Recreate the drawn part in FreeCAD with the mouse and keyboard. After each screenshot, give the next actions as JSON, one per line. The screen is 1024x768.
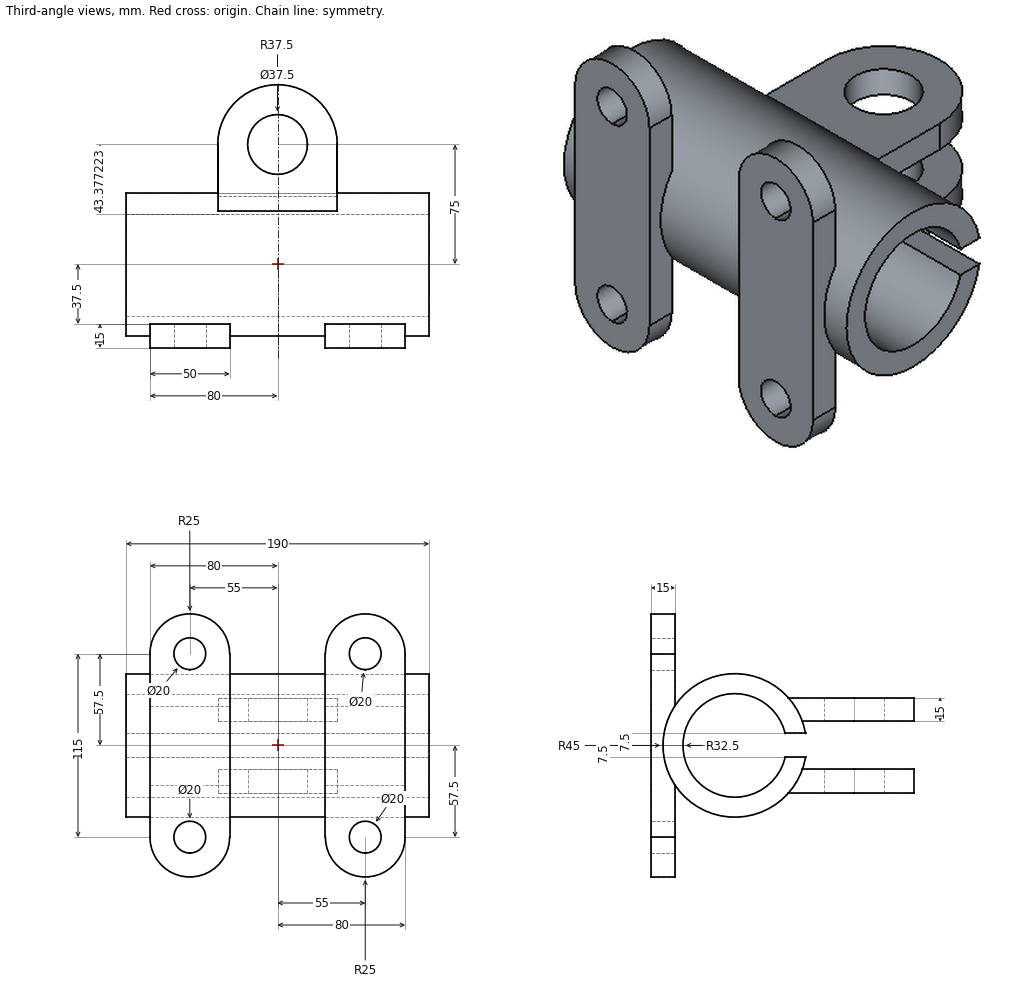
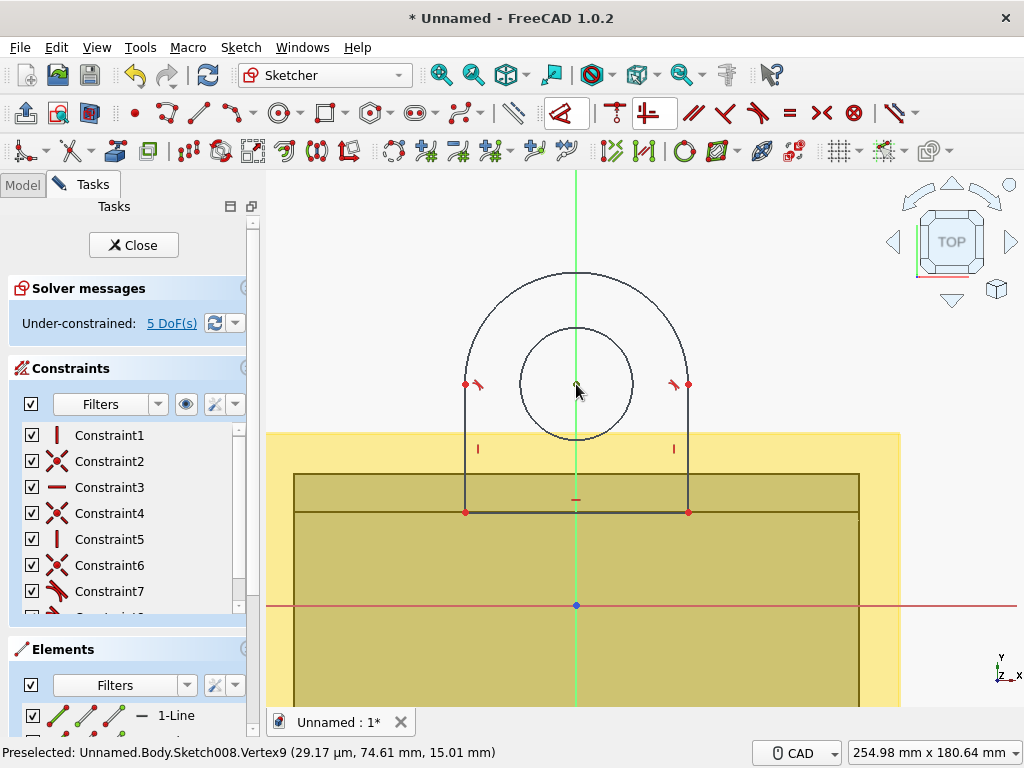
{"action": "left_click", "coordinate": [576, 645]}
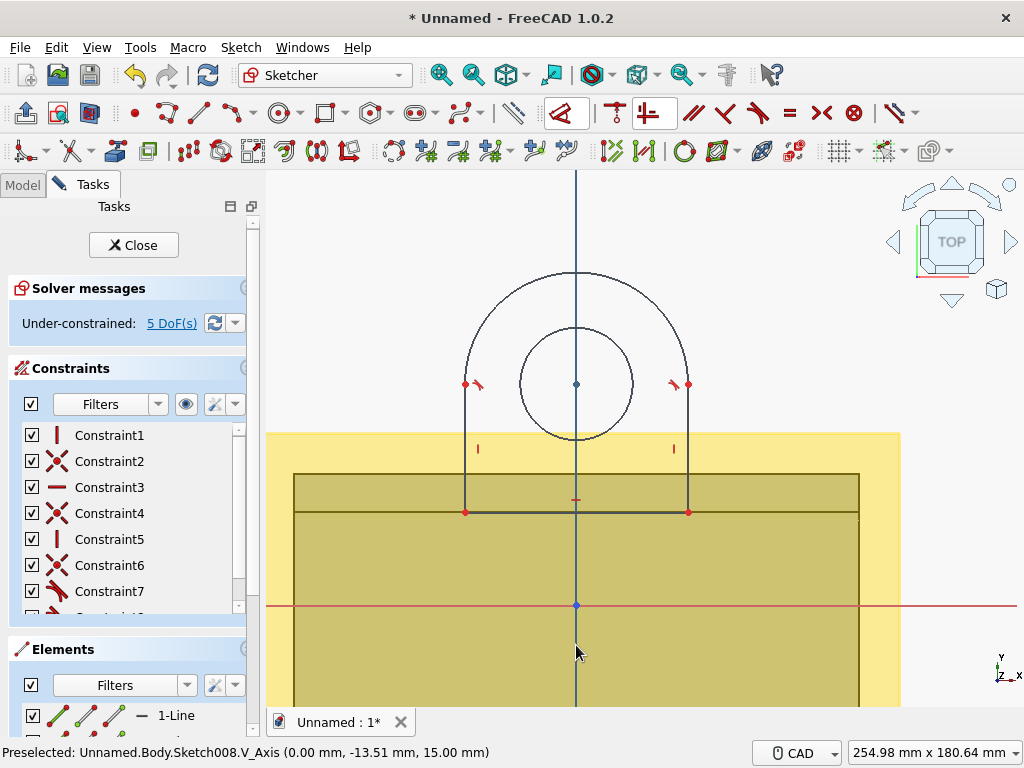
{"action": "left_click", "coordinate": [616, 114]}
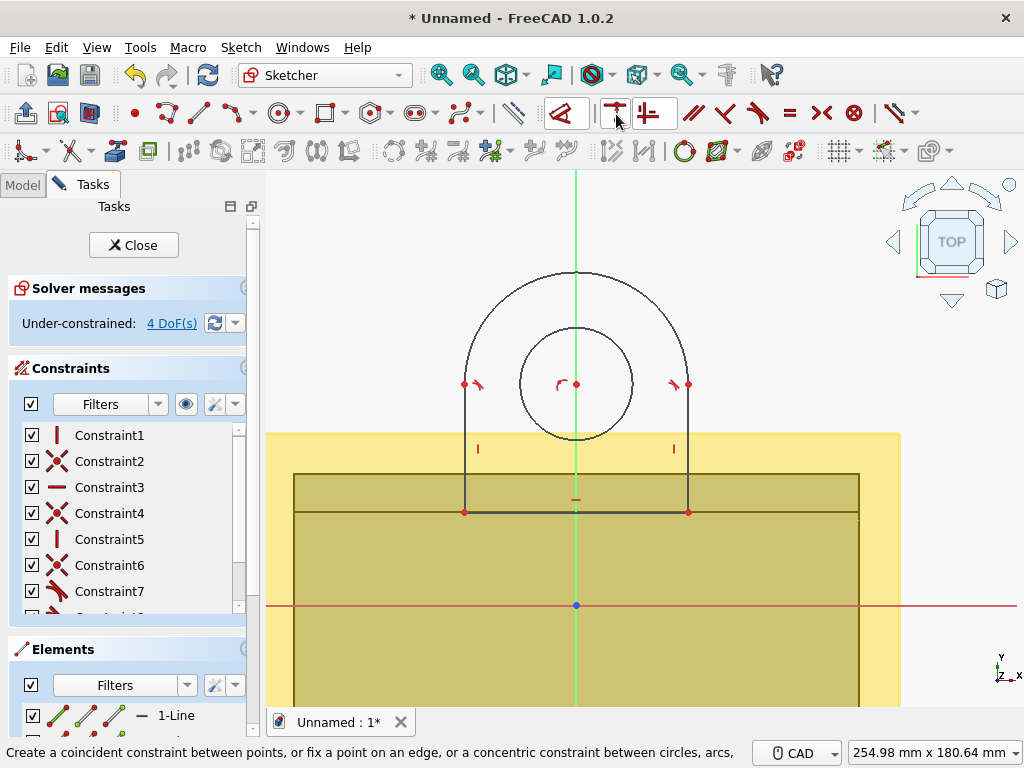
{"action": "left_click", "coordinate": [642, 294]}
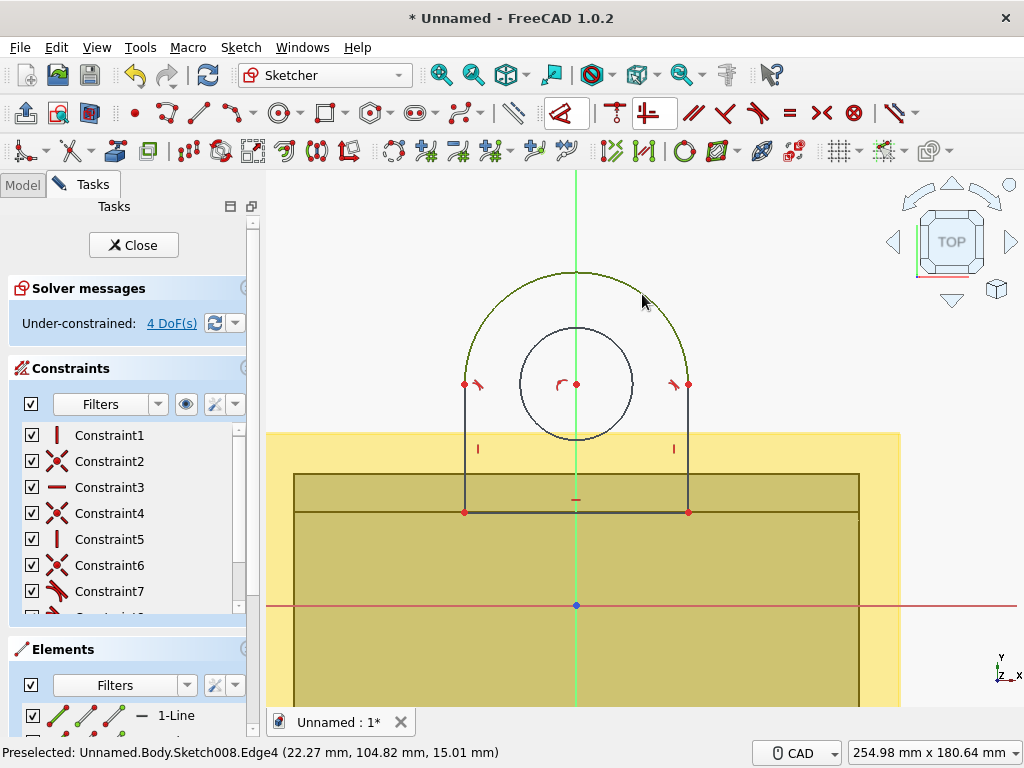
{"action": "left_click", "coordinate": [584, 114]}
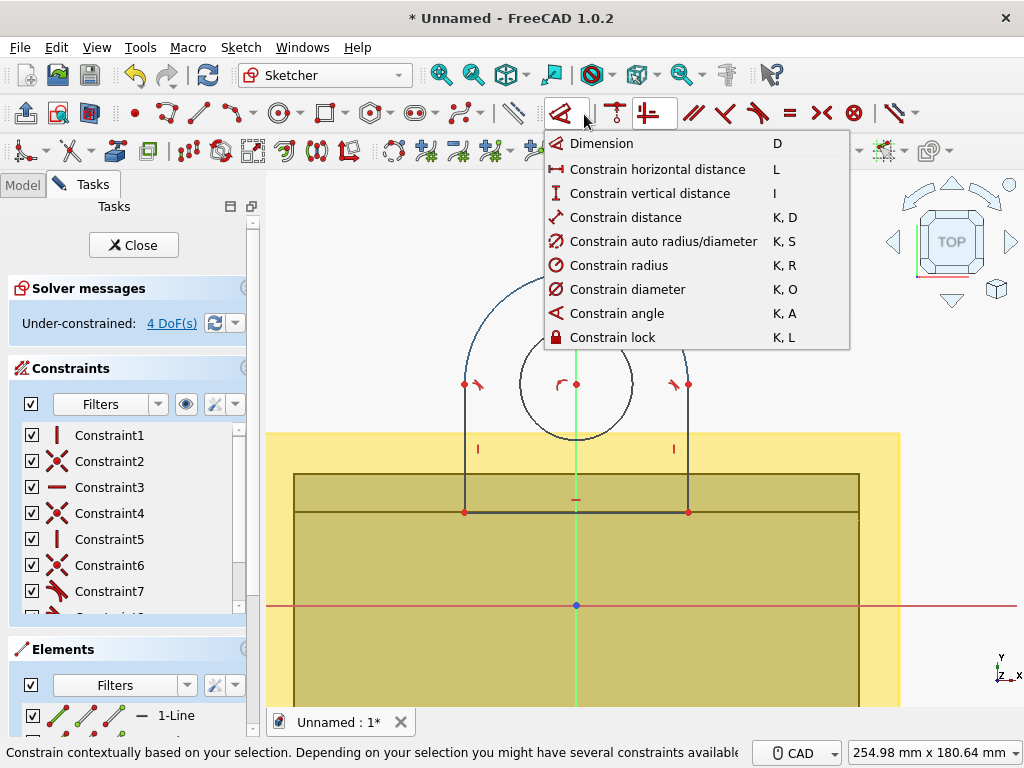
{"action": "left_click", "coordinate": [697, 265]}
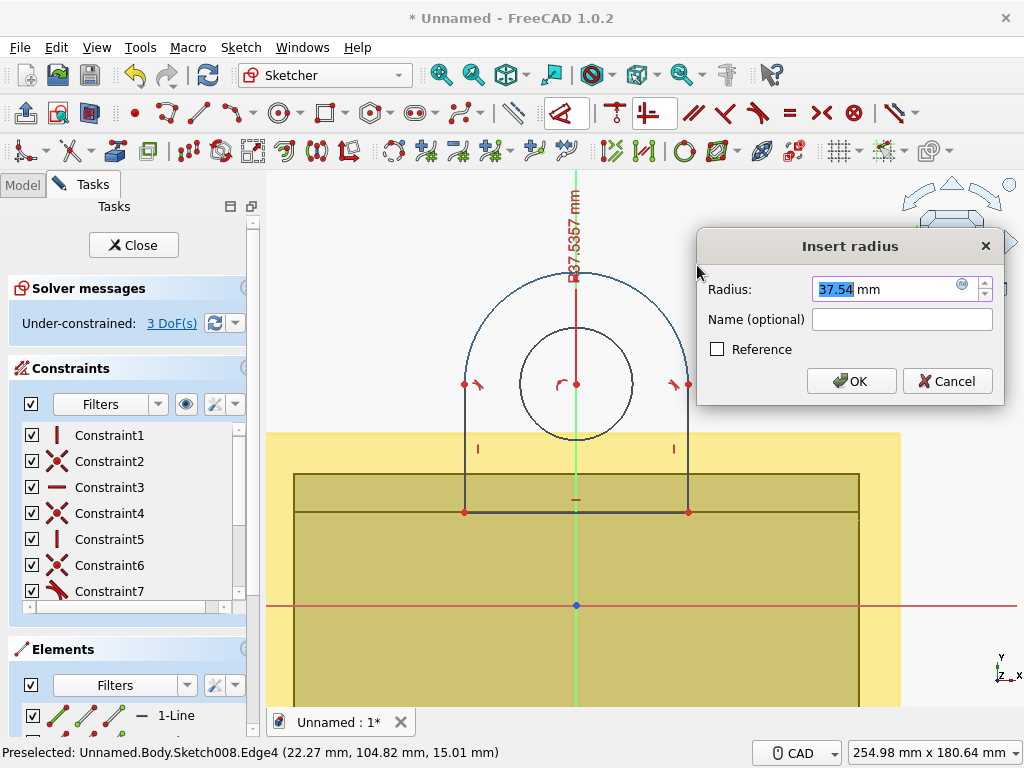
{"action": "type", "text": "37.5"}
{"action": "key", "text": "Return"}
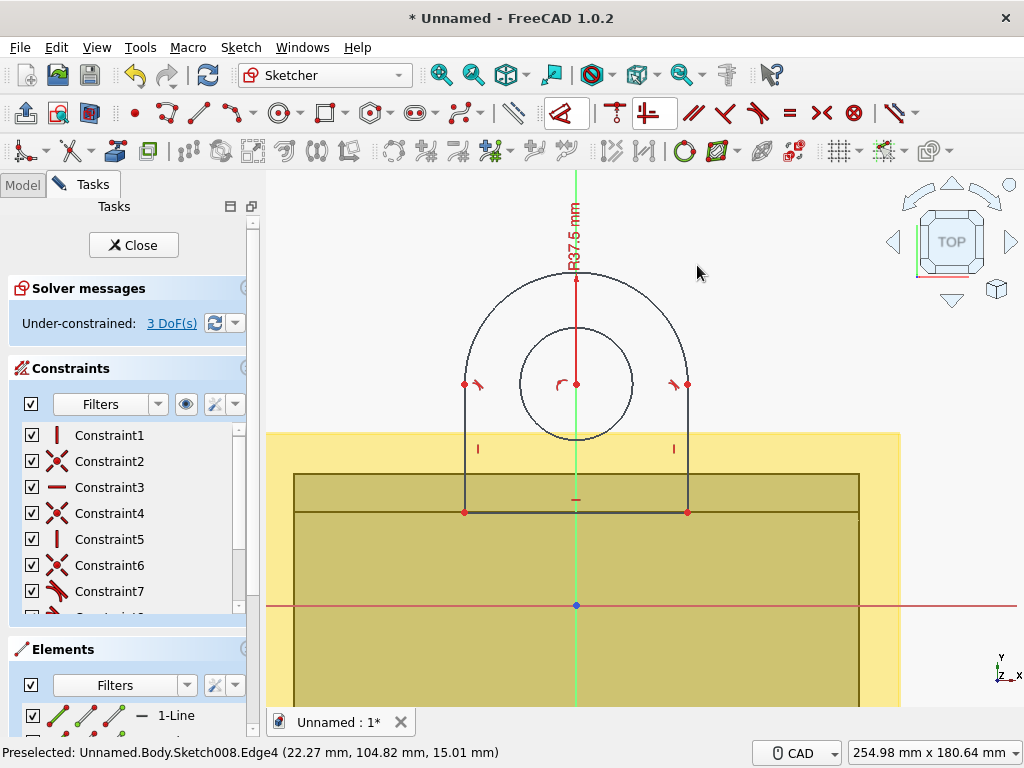
{"action": "left_click", "coordinate": [616, 344]}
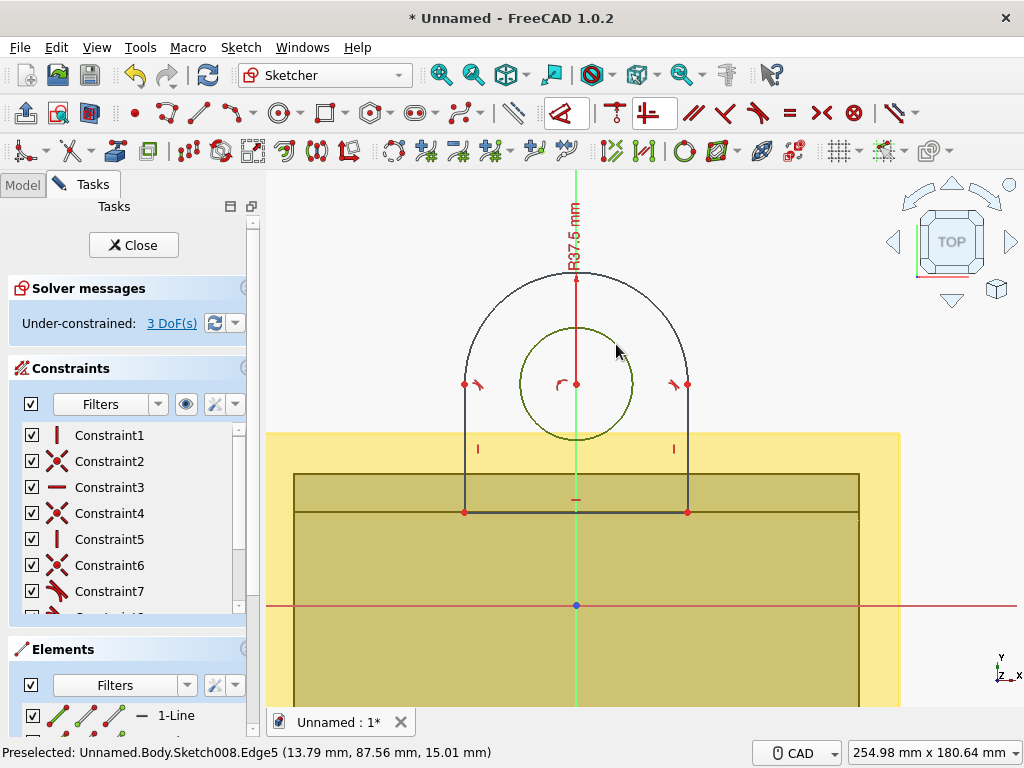
{"action": "left_click", "coordinate": [584, 114]}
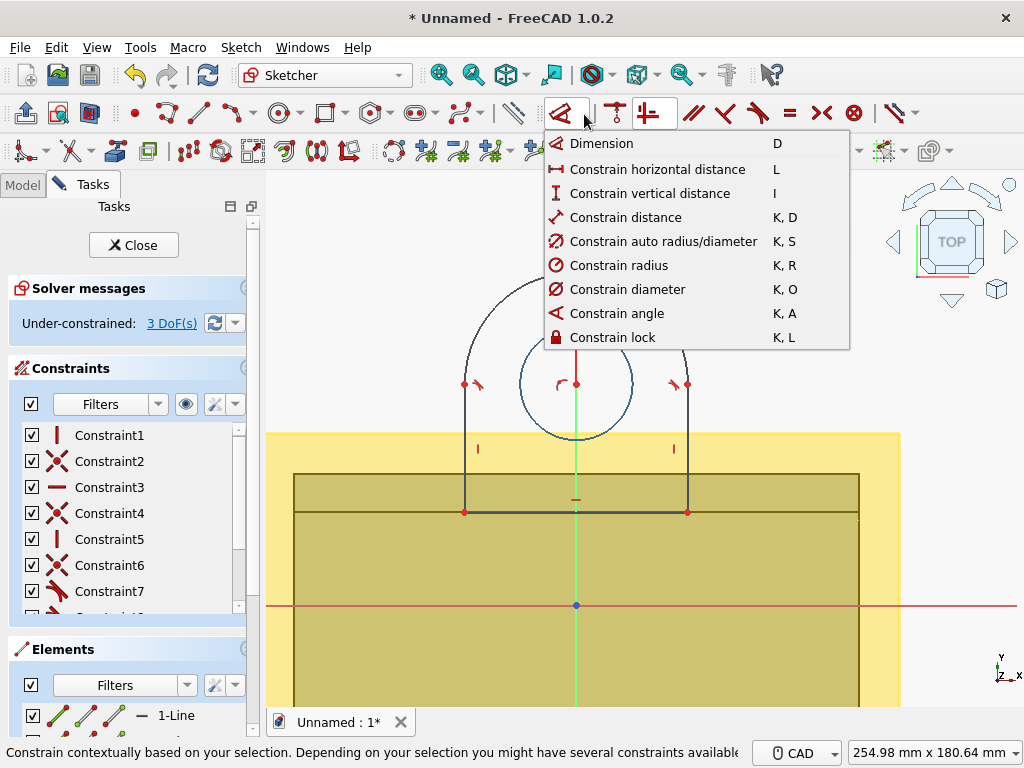
{"action": "left_click", "coordinate": [697, 289]}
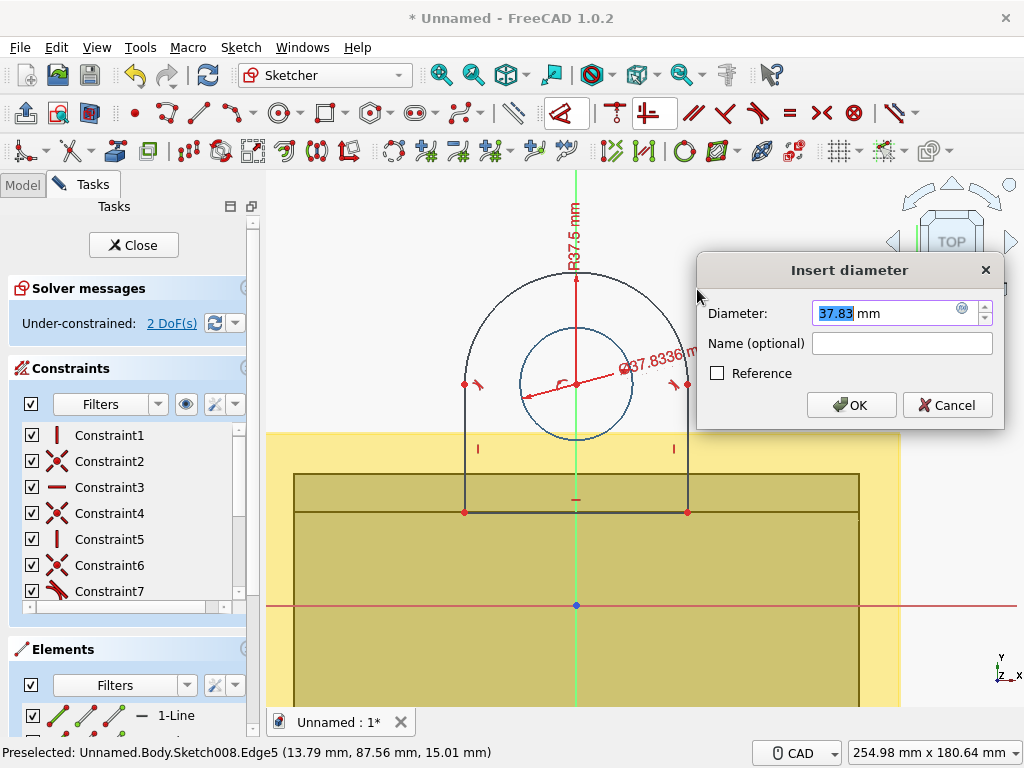
{"action": "type", "text": "37.5"}
{"action": "key", "text": "Return"}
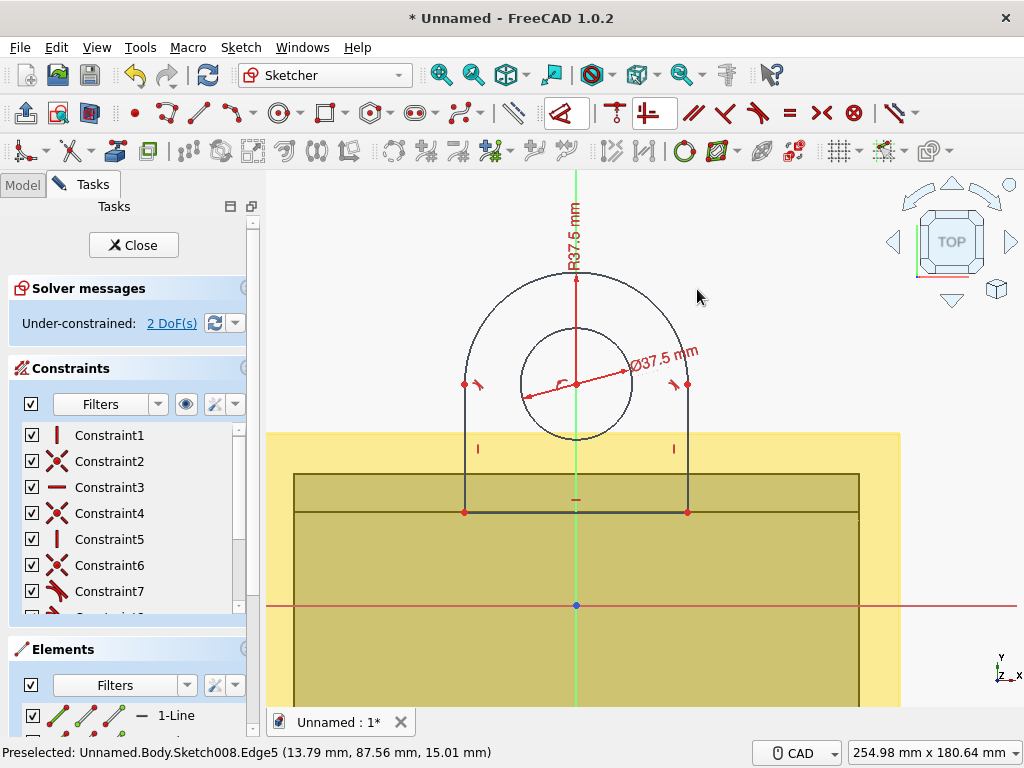
{"action": "left_click", "coordinate": [576, 384]}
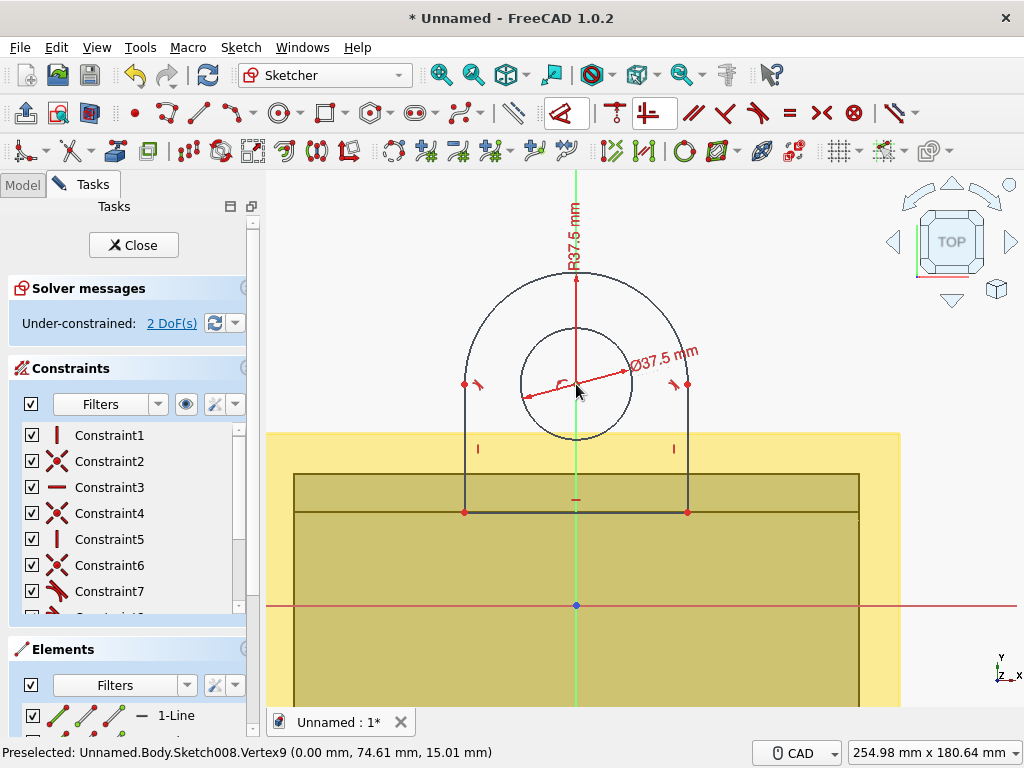
{"action": "left_click", "coordinate": [584, 114]}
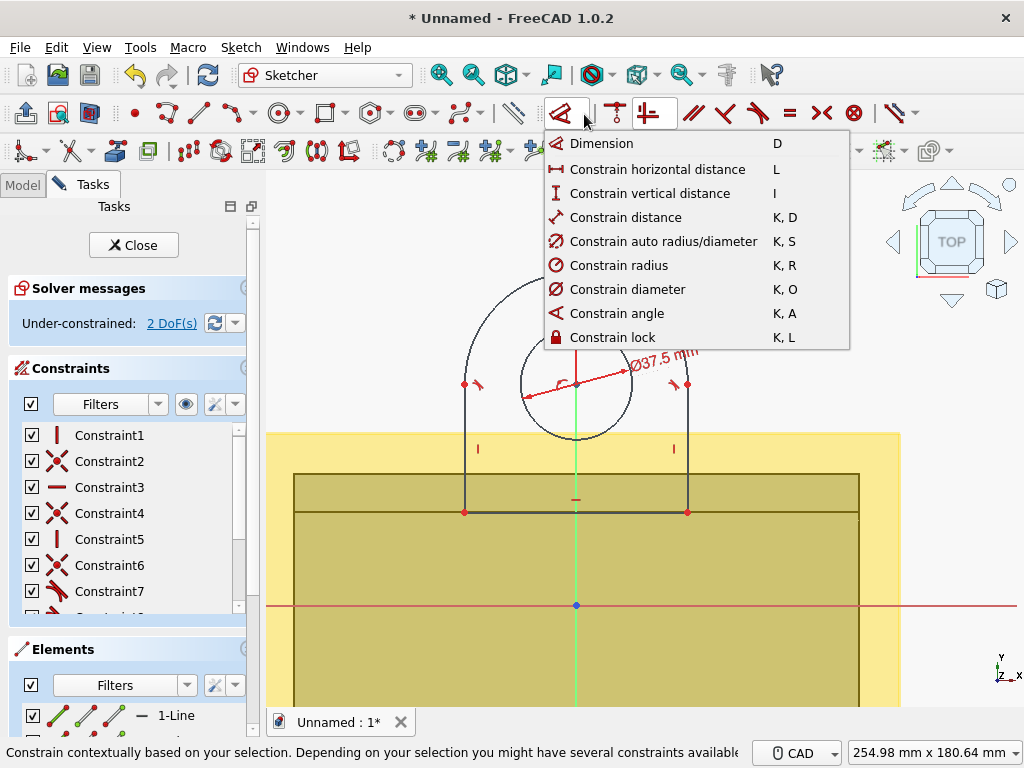
{"action": "left_click", "coordinate": [697, 193]}